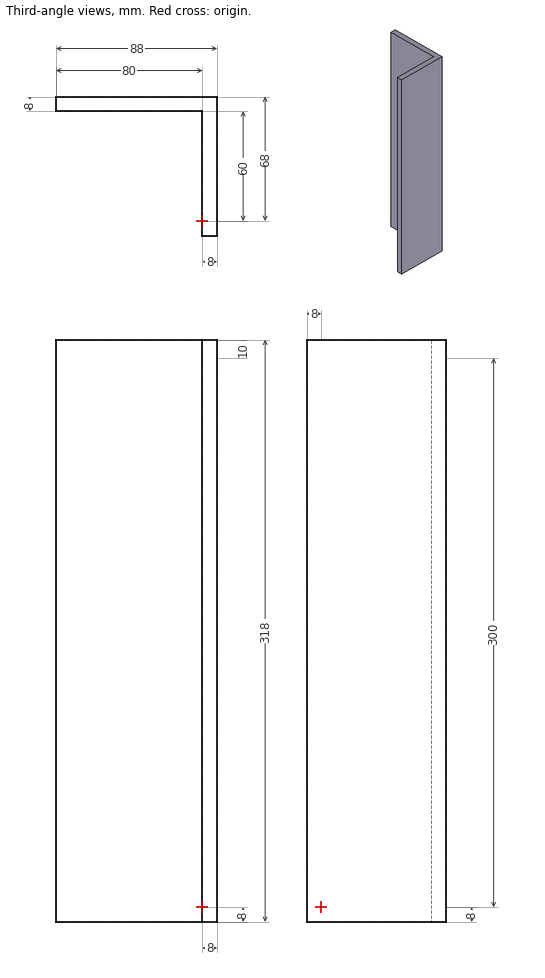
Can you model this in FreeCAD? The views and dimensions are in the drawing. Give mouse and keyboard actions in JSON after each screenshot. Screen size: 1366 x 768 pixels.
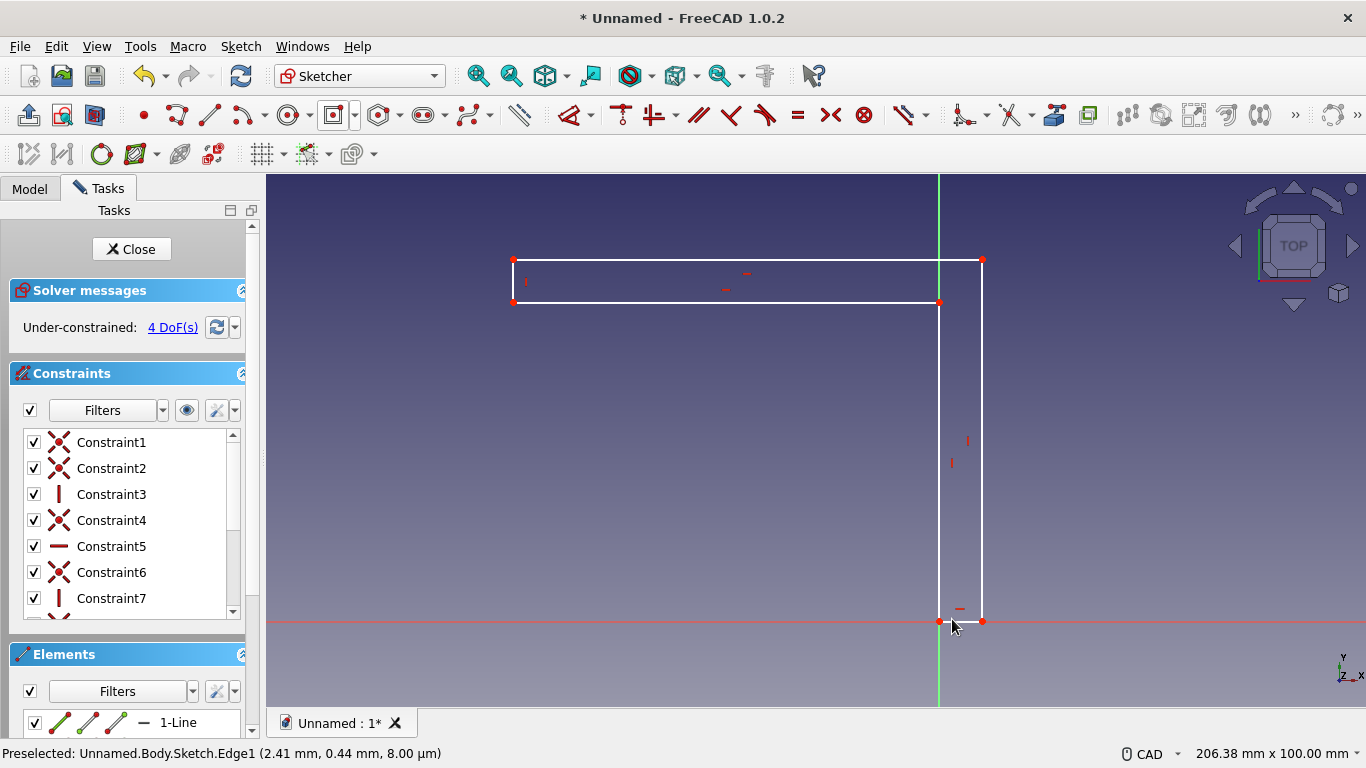
{"action": "left_click", "coordinate": [568, 116]}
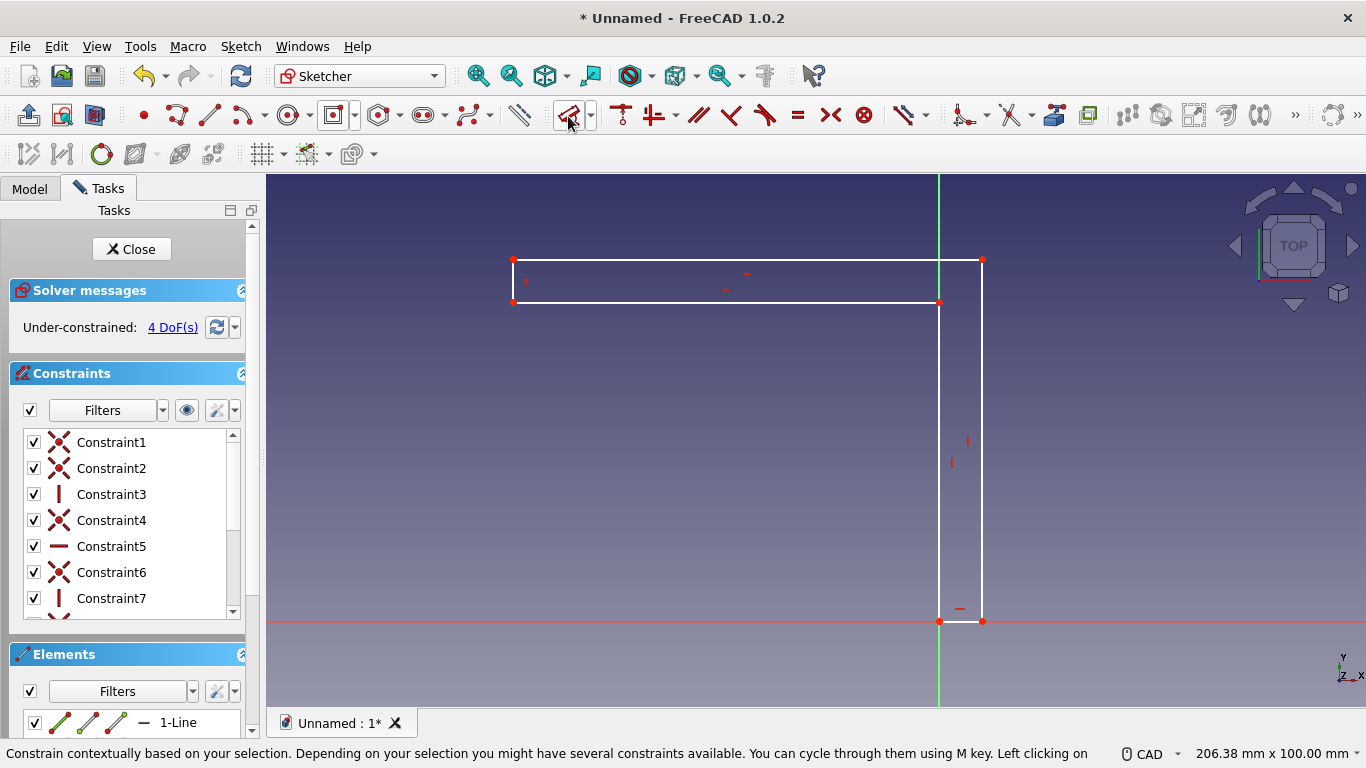
{"action": "left_click", "coordinate": [952, 622]}
{"action": "left_click", "coordinate": [961, 656]}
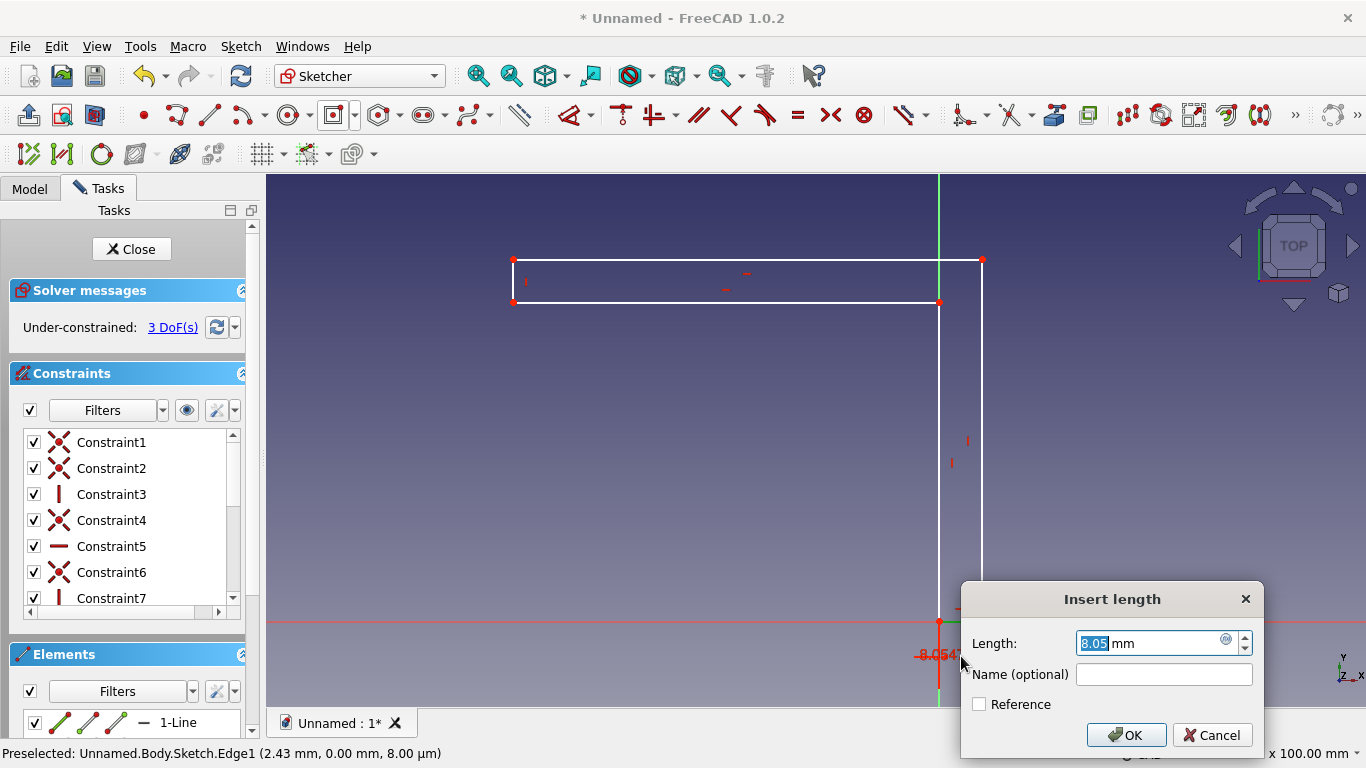
{"action": "type", "text": "8"}
{"action": "key", "text": "Return"}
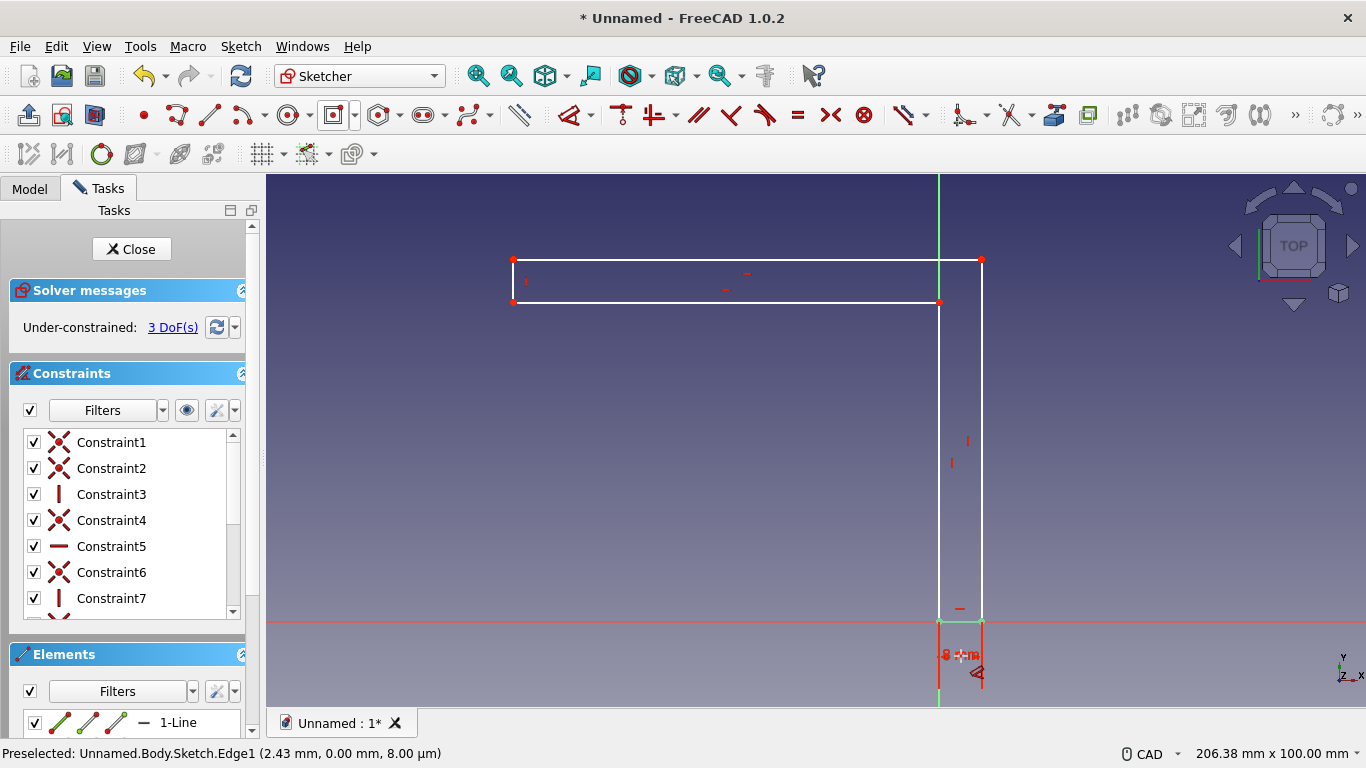
{"action": "left_click", "coordinate": [513, 273]}
{"action": "left_click", "coordinate": [479, 281]}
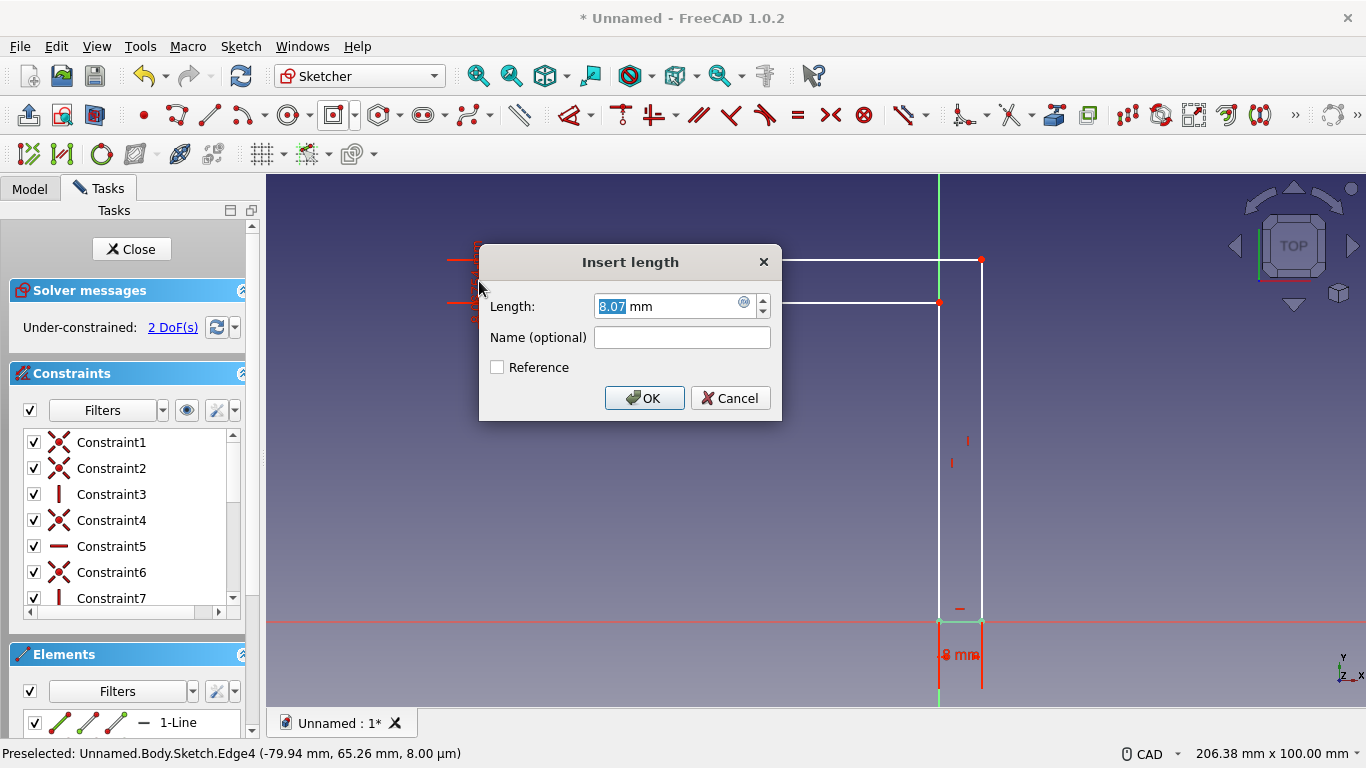
{"action": "type", "text": "8"}
{"action": "key", "text": "Return"}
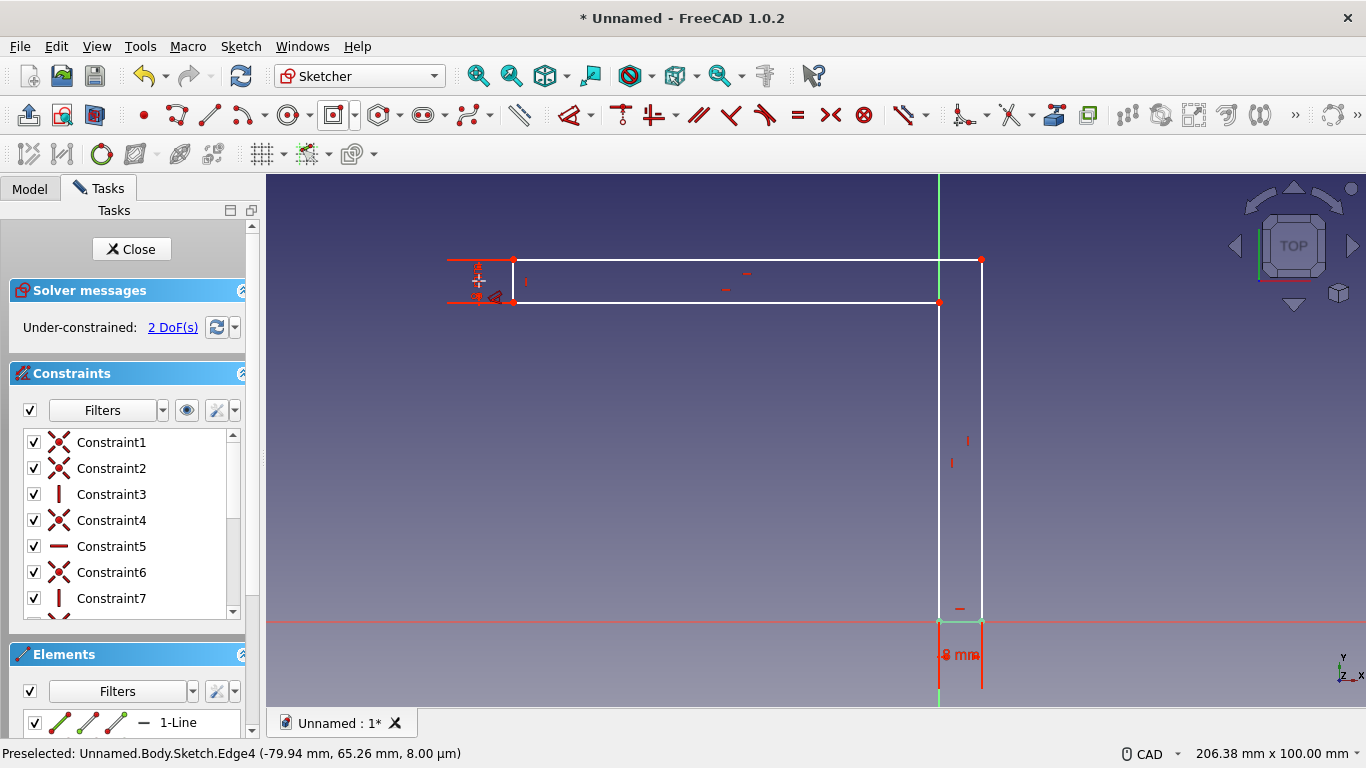
{"action": "left_click", "coordinate": [982, 513]}
{"action": "left_click", "coordinate": [1016, 441]}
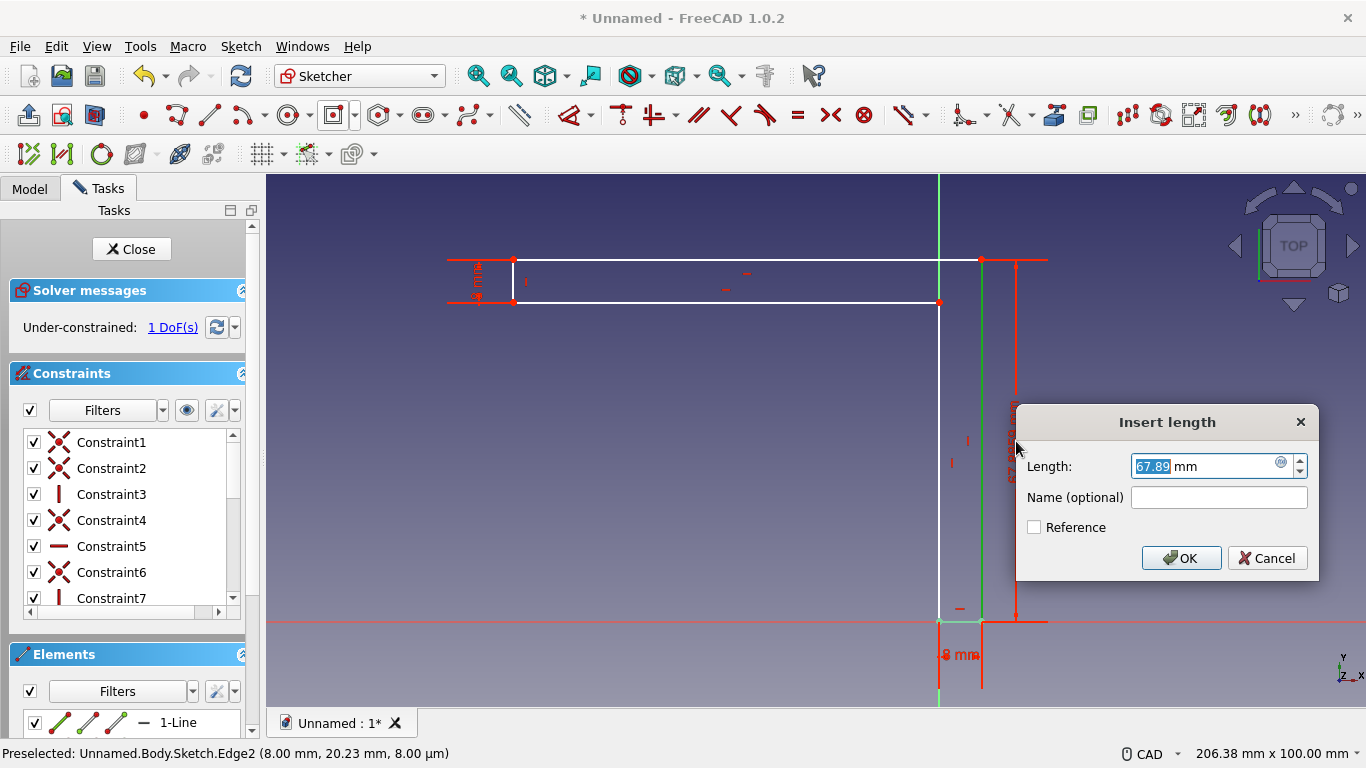
{"action": "type", "text": "68"}
{"action": "key", "text": "Return"}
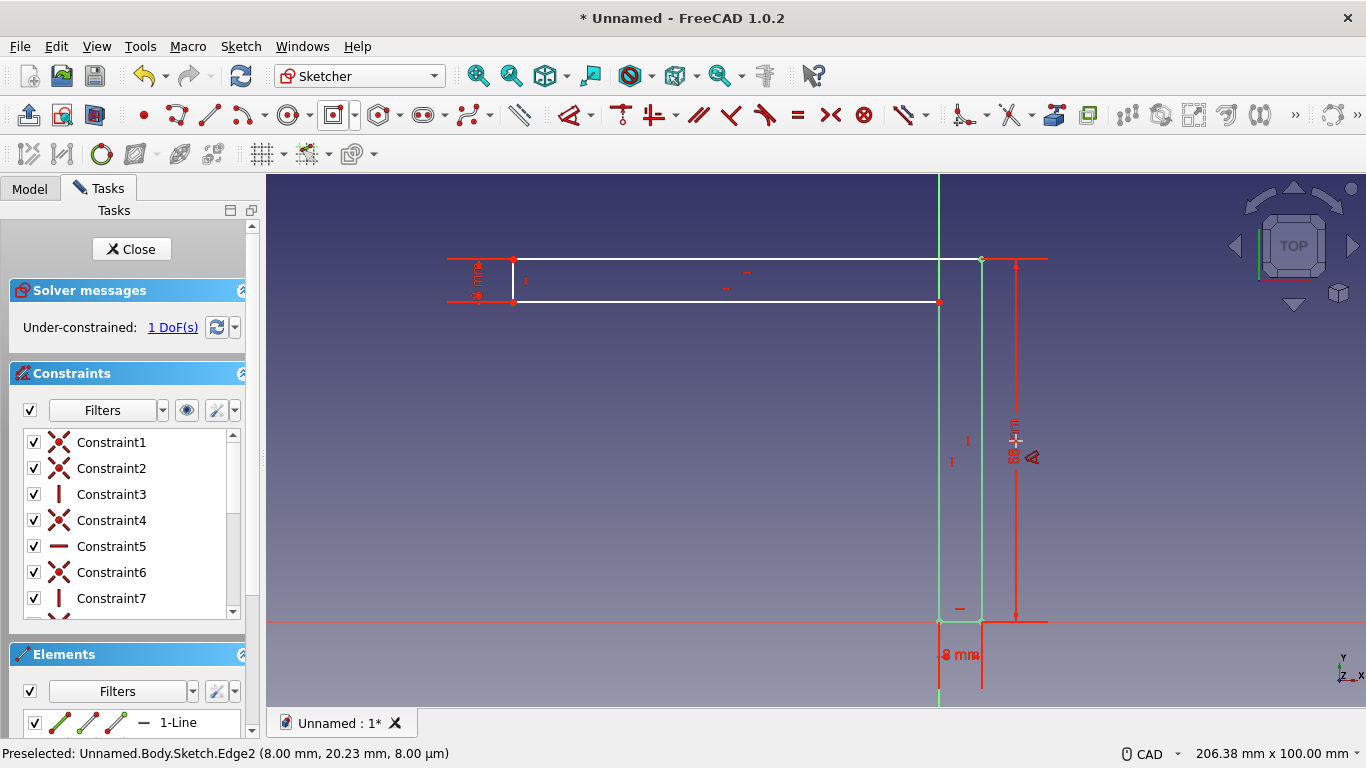
{"action": "left_click", "coordinate": [841, 259]}
{"action": "left_click", "coordinate": [747, 225]}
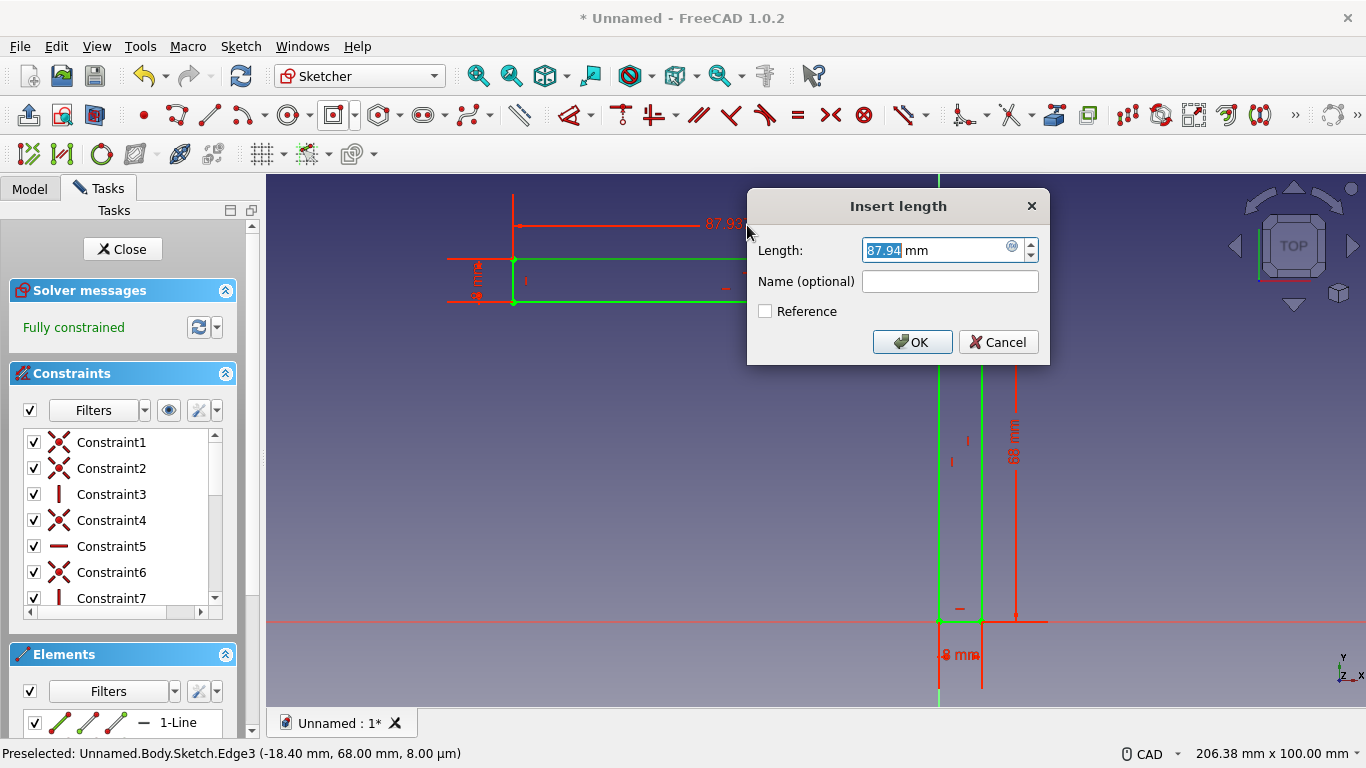
{"action": "type", "text": "88"}
{"action": "key", "text": "Return"}
{"action": "key", "text": "Escape"}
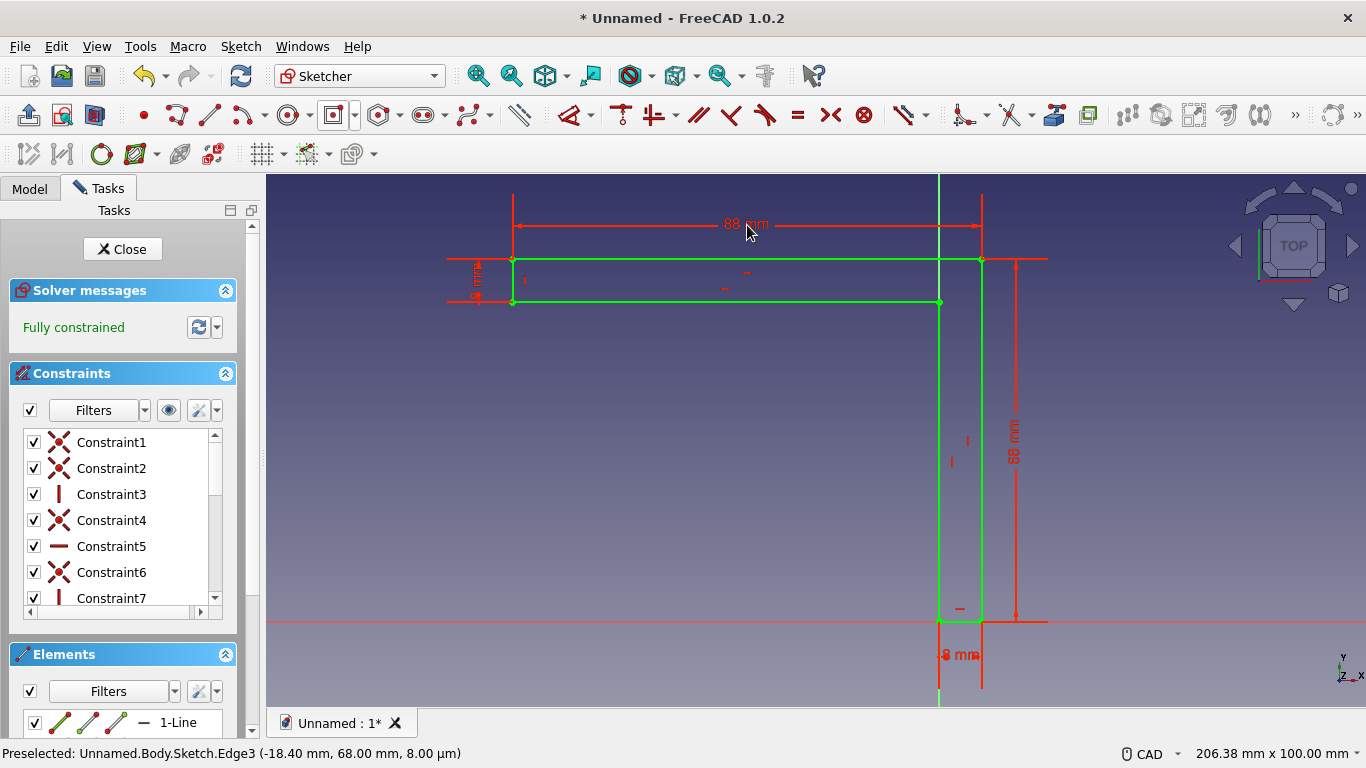
{"action": "left_click", "coordinate": [123, 249]}